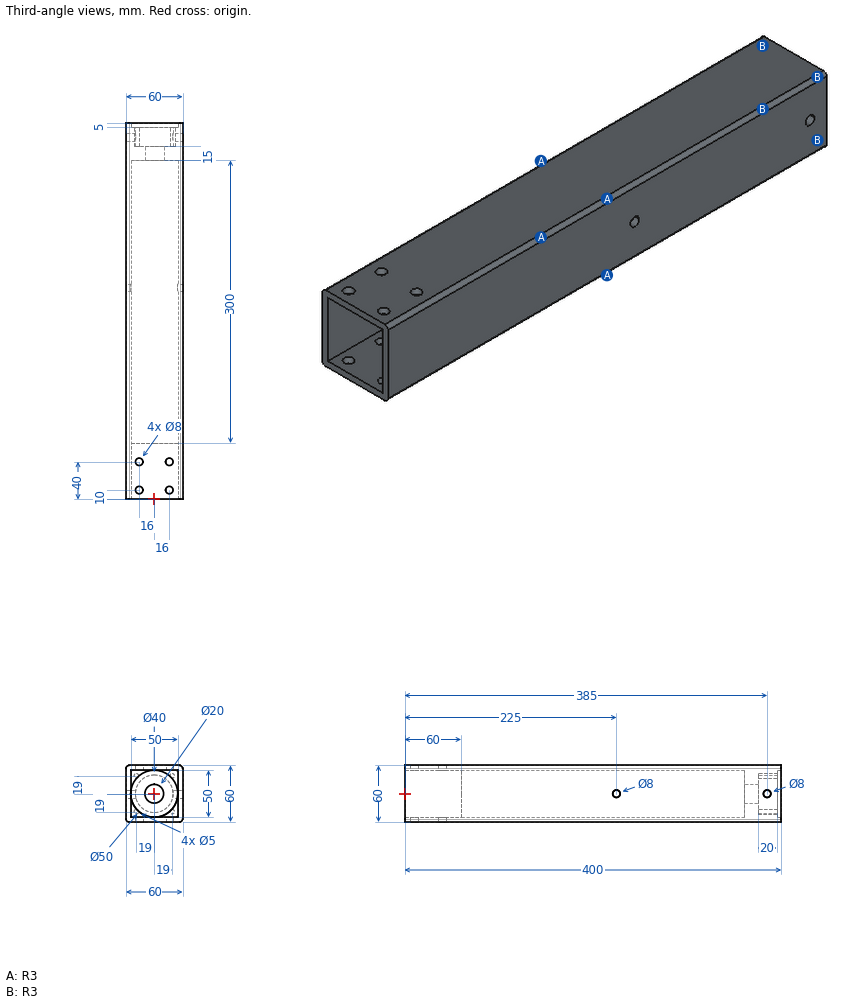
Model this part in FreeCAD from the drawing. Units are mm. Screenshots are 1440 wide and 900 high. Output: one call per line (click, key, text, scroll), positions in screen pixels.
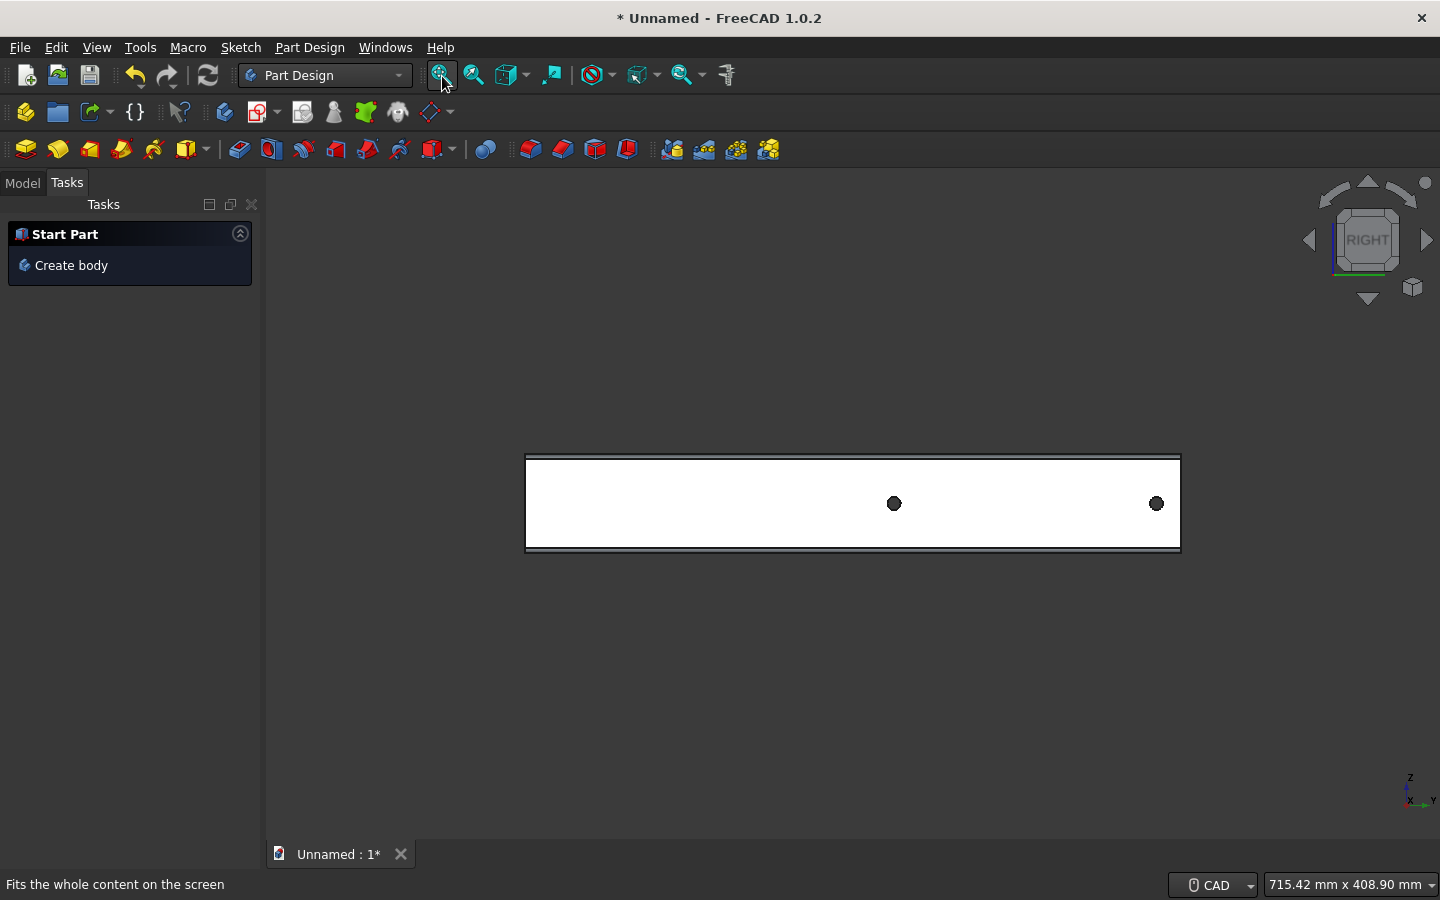
key(5)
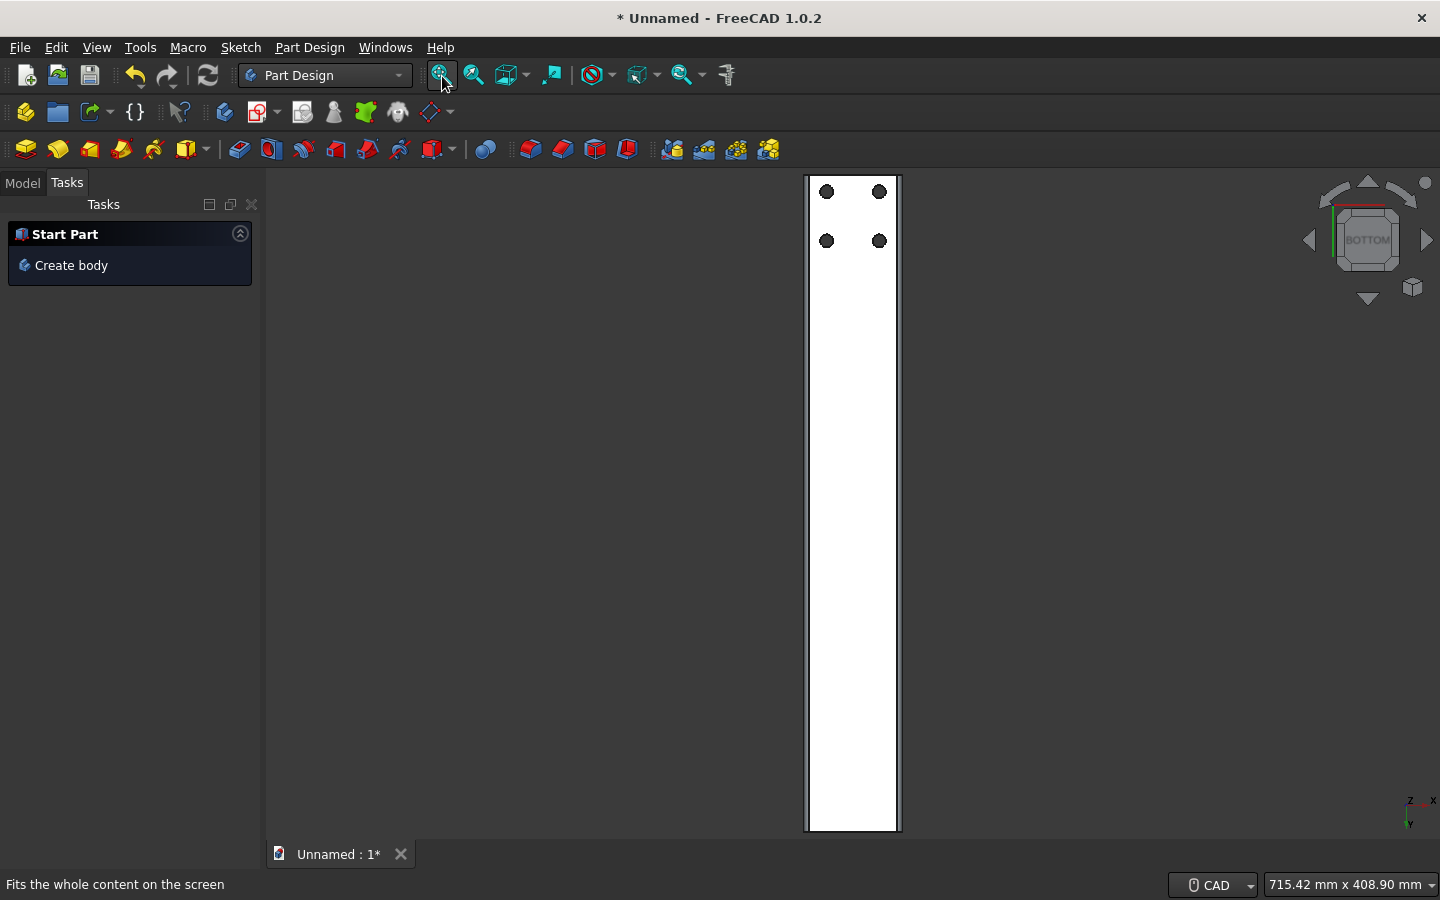
key(4)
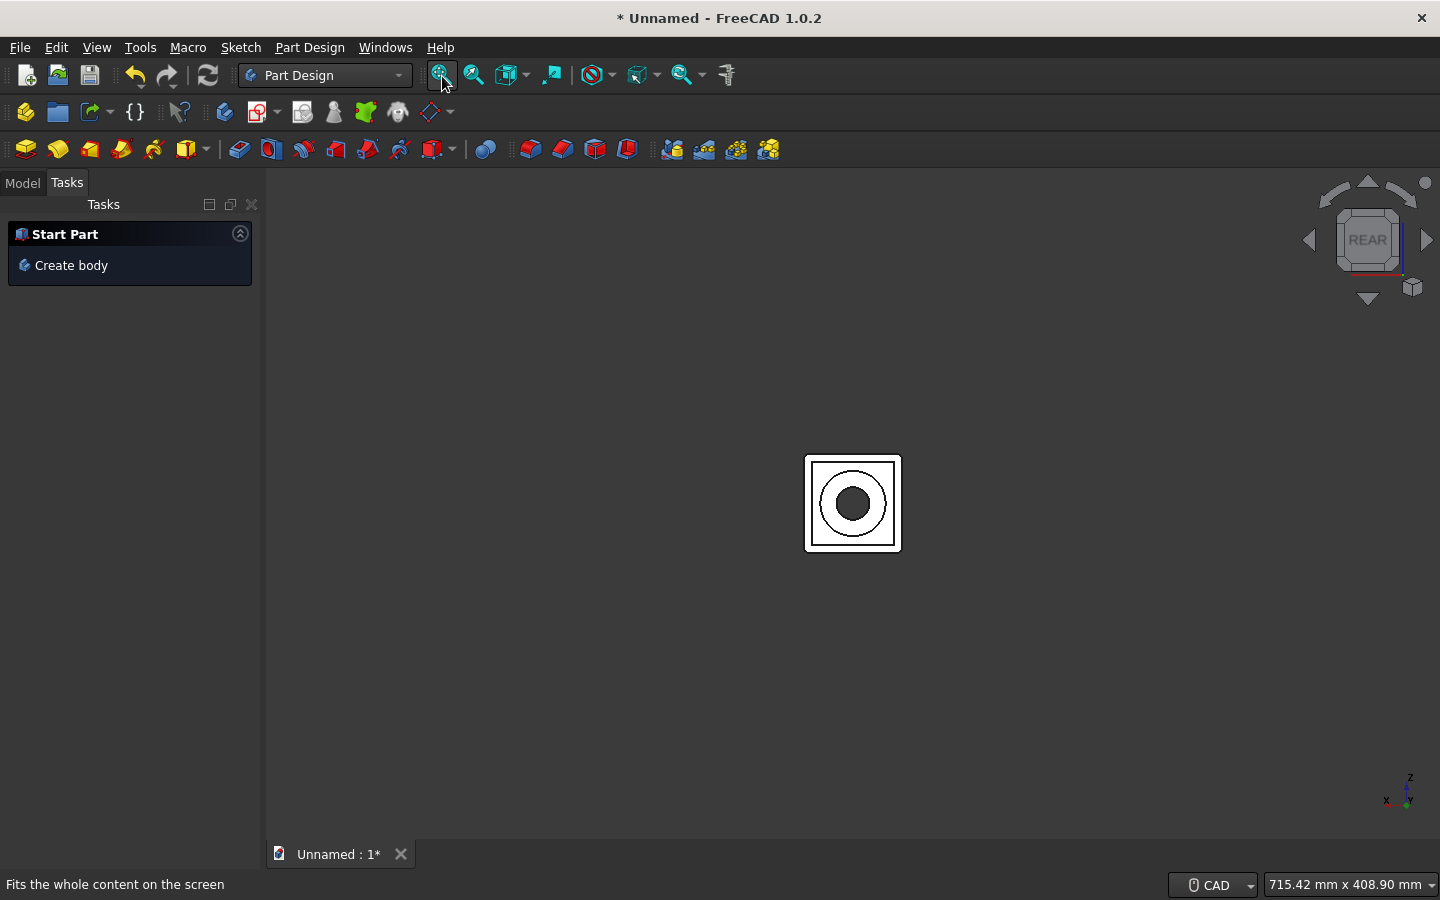
key(v)
key(f)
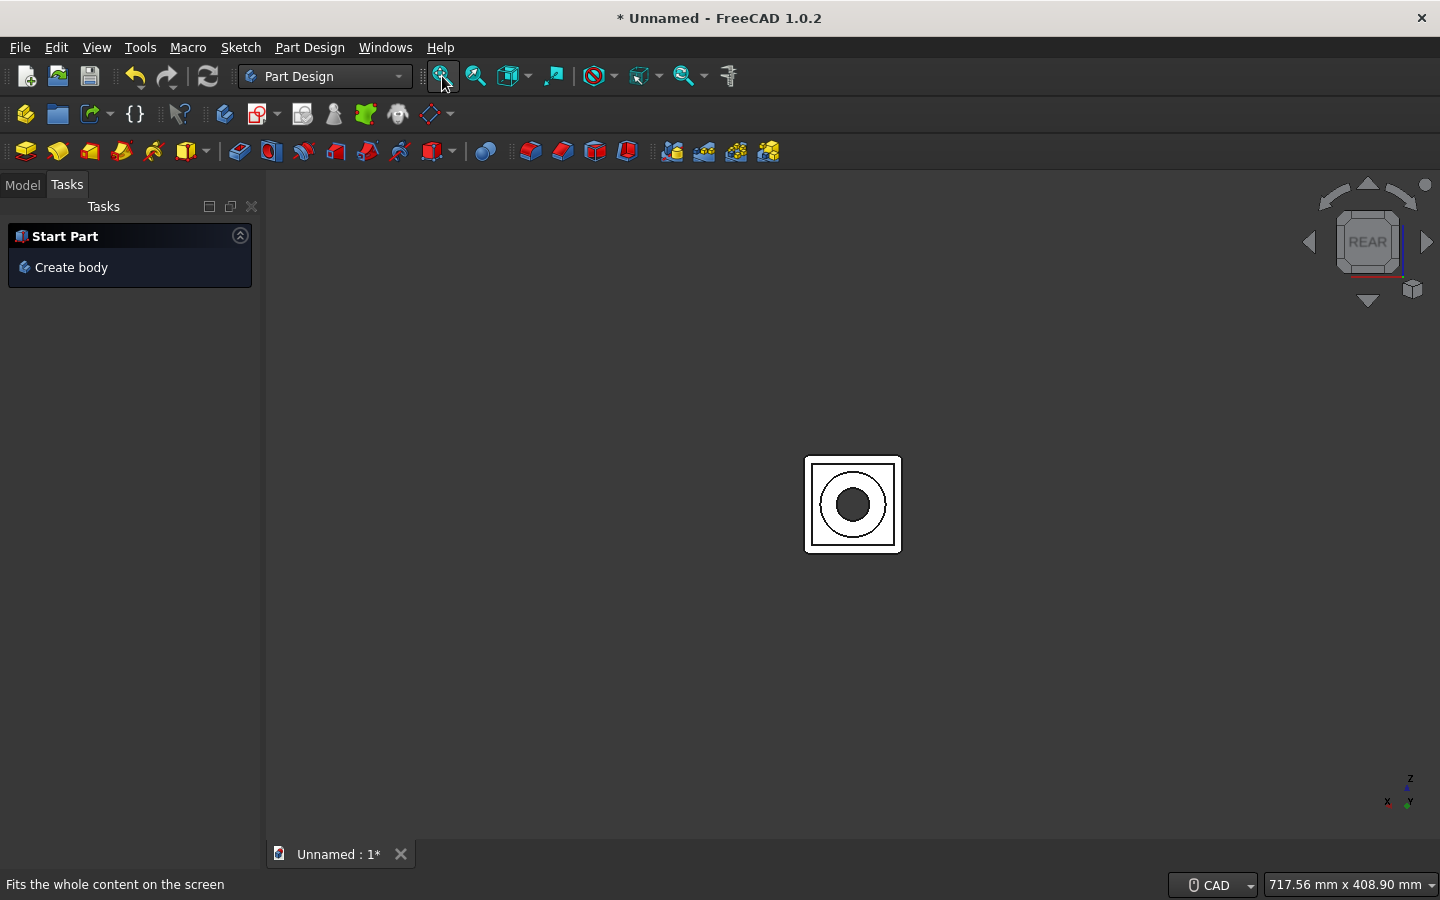
scroll(812, 544, up, 8)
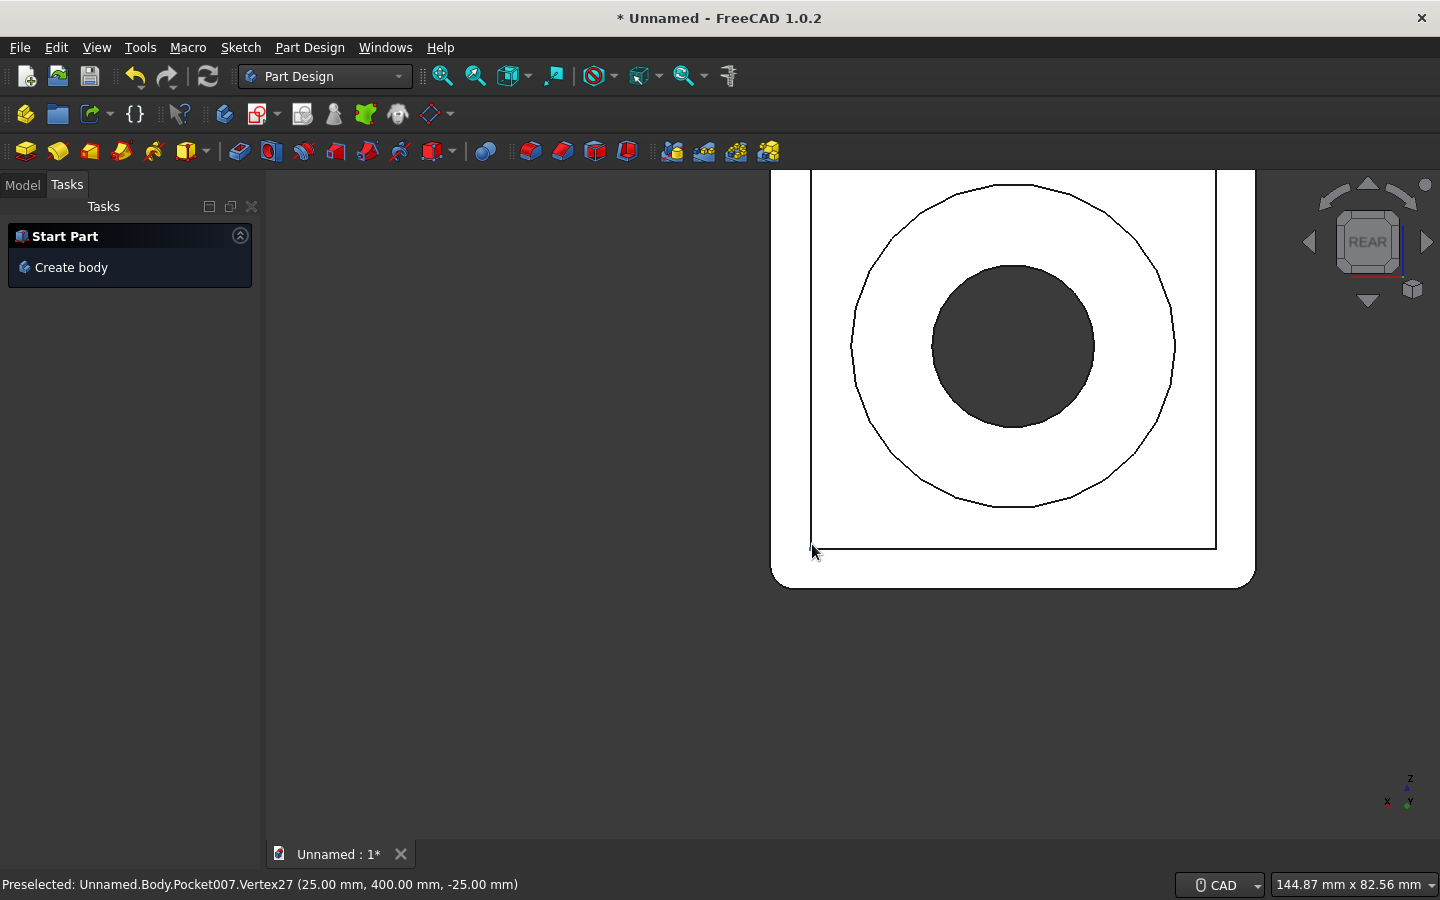
key(v)
key(f)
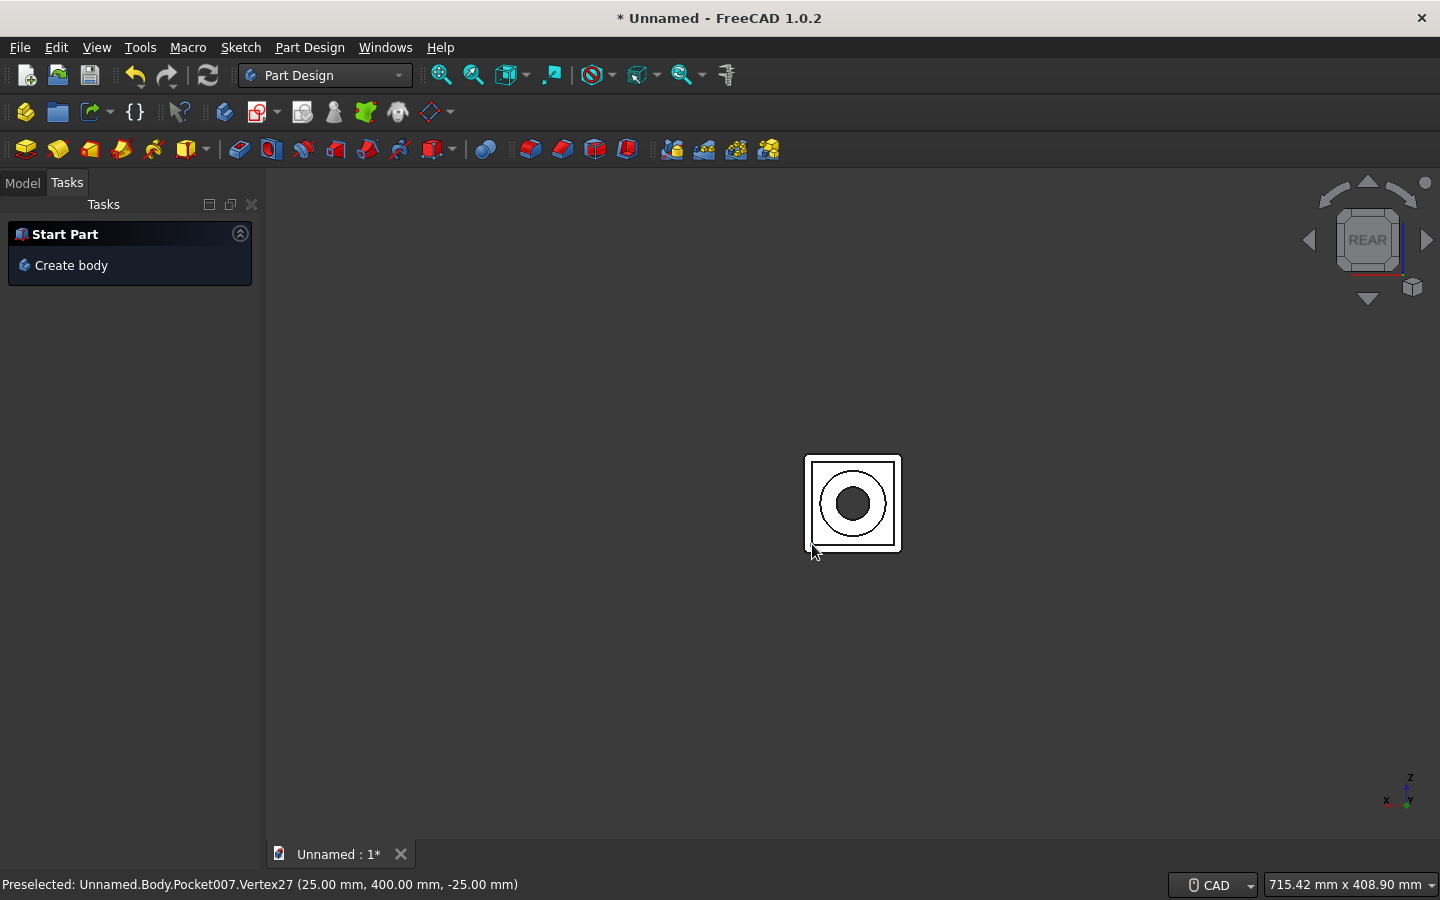
key(6)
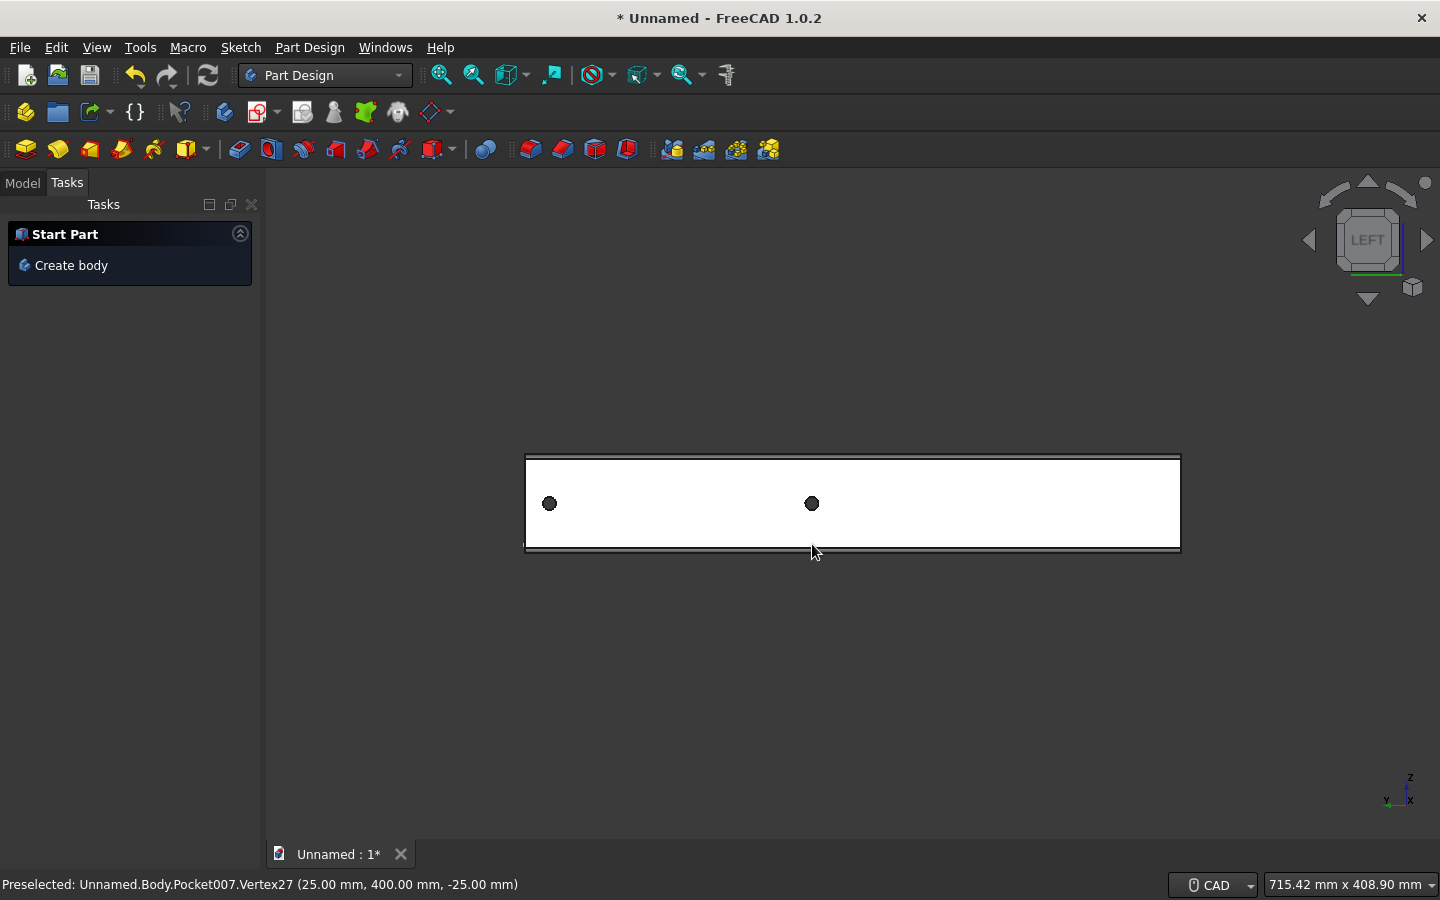
scroll(529, 544, up, 8)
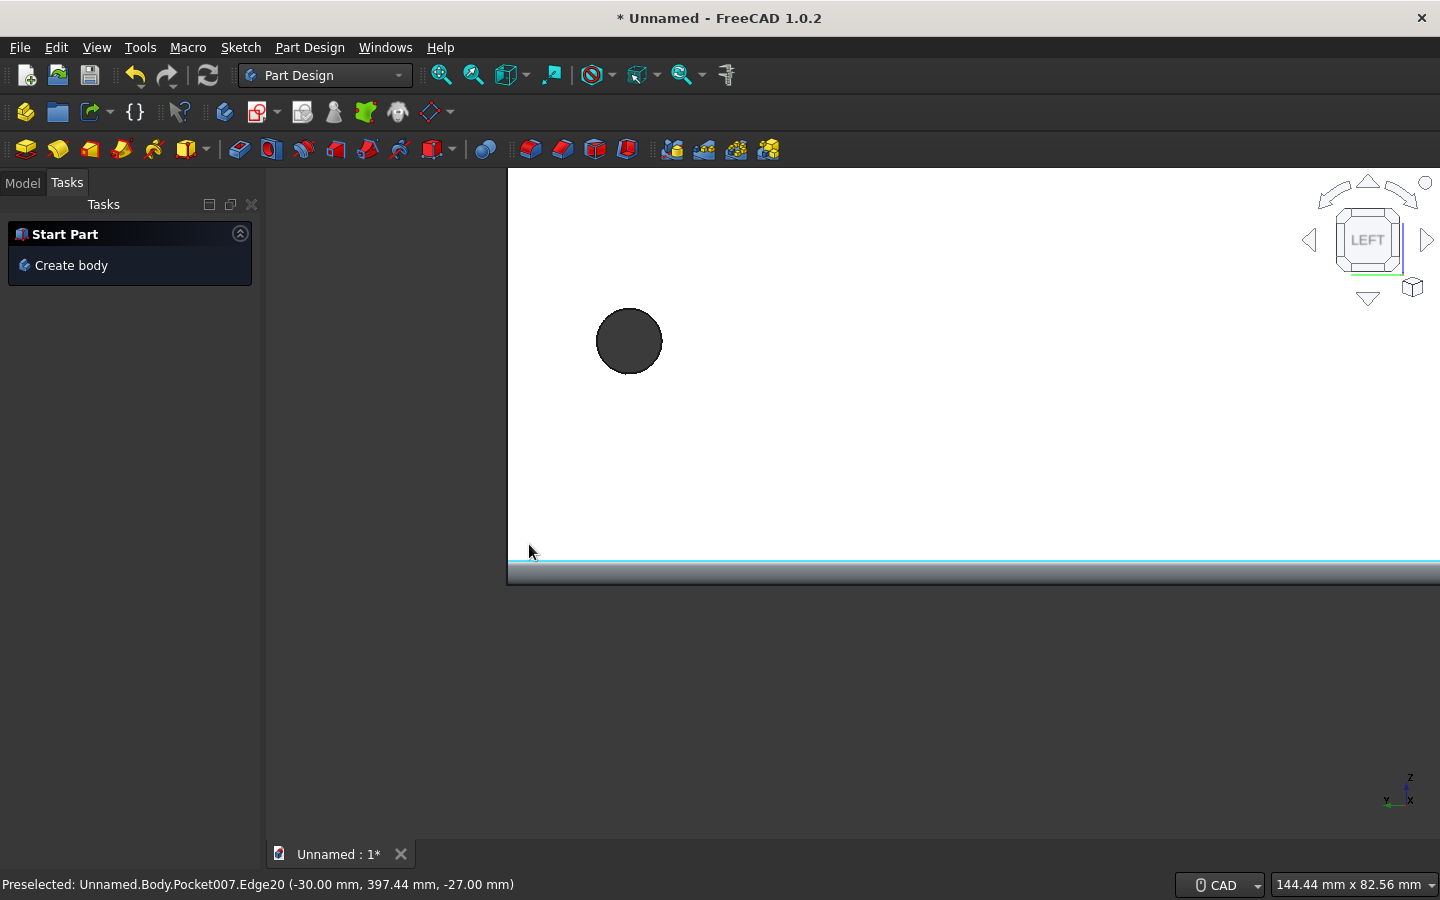
click(442, 76)